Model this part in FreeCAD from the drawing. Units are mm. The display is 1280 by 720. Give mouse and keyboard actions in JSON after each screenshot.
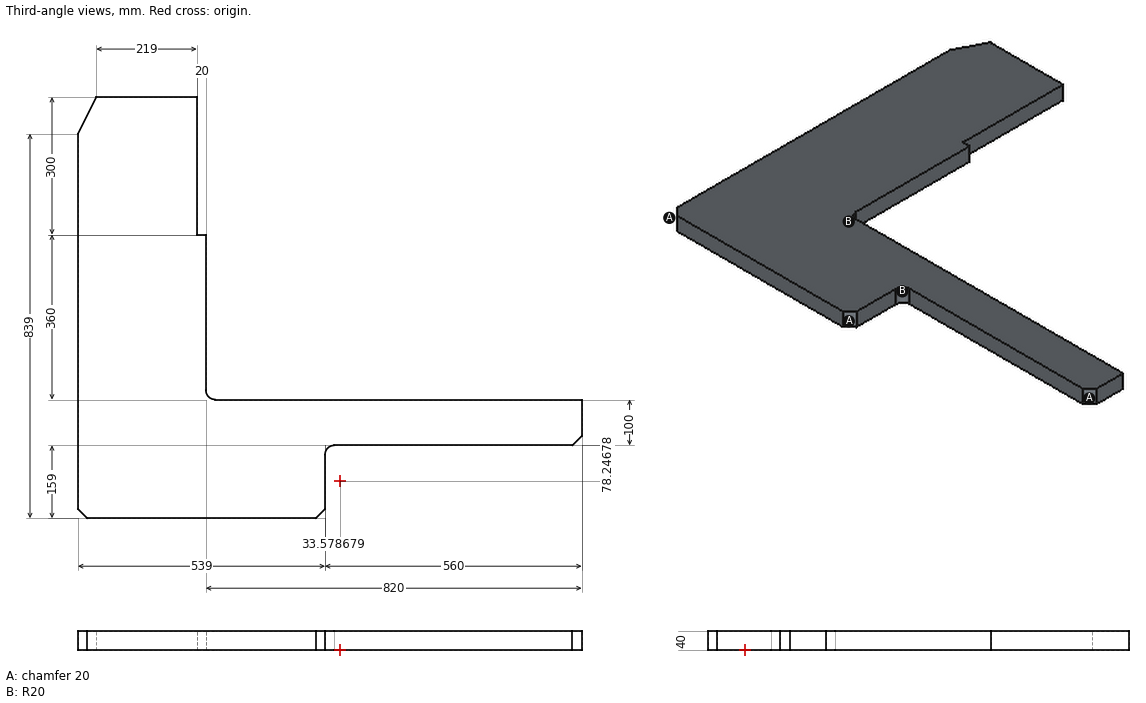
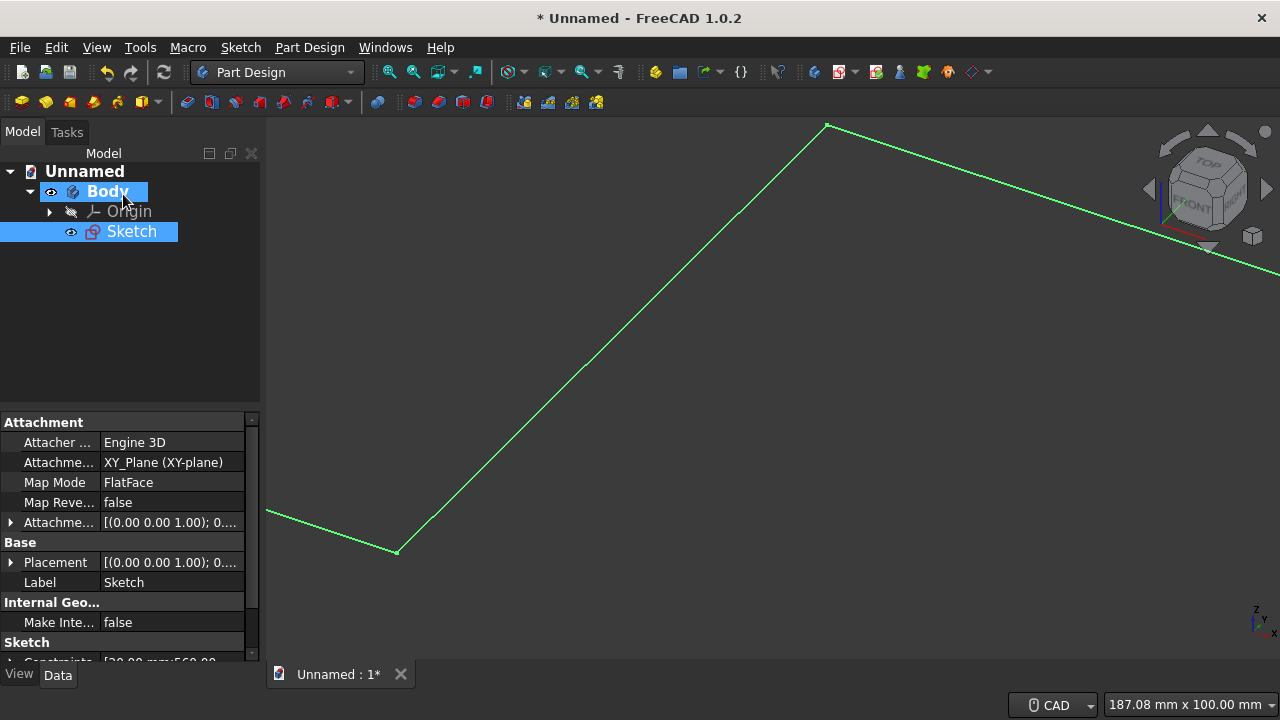
{"action": "left_click", "coordinate": [22, 102]}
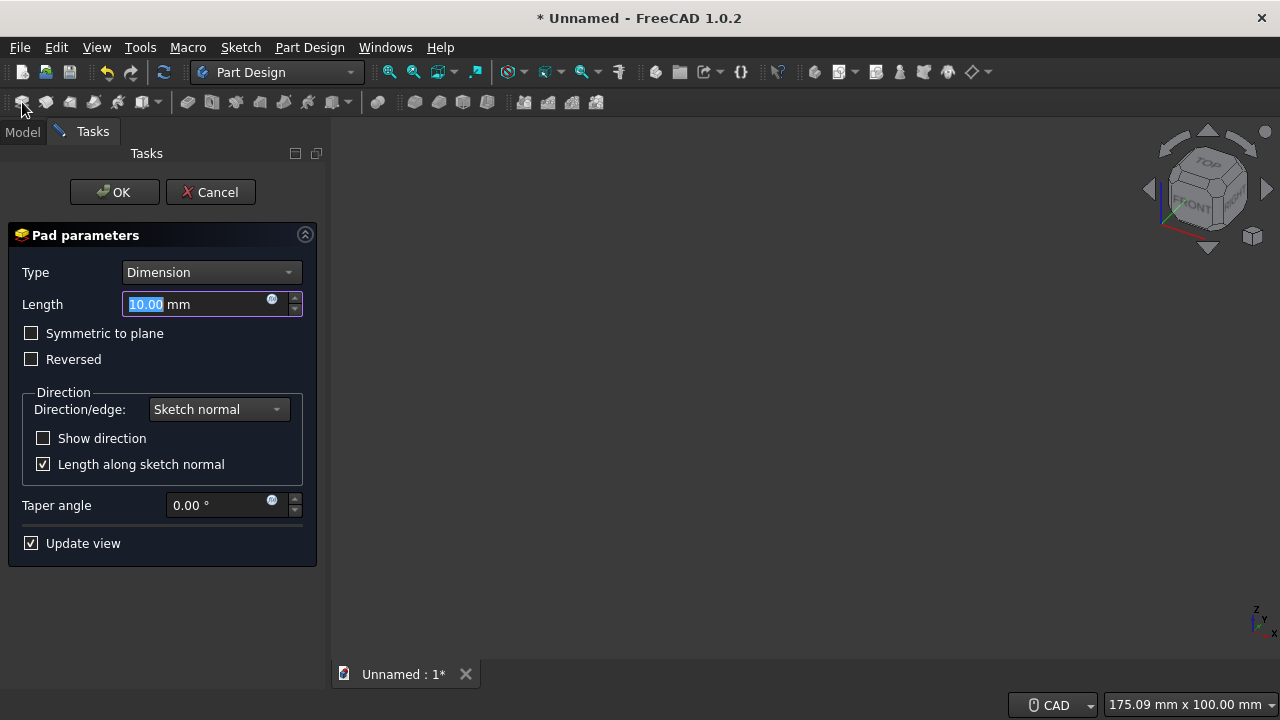
{"action": "type", "text": "40"}
{"action": "key", "text": "Tab"}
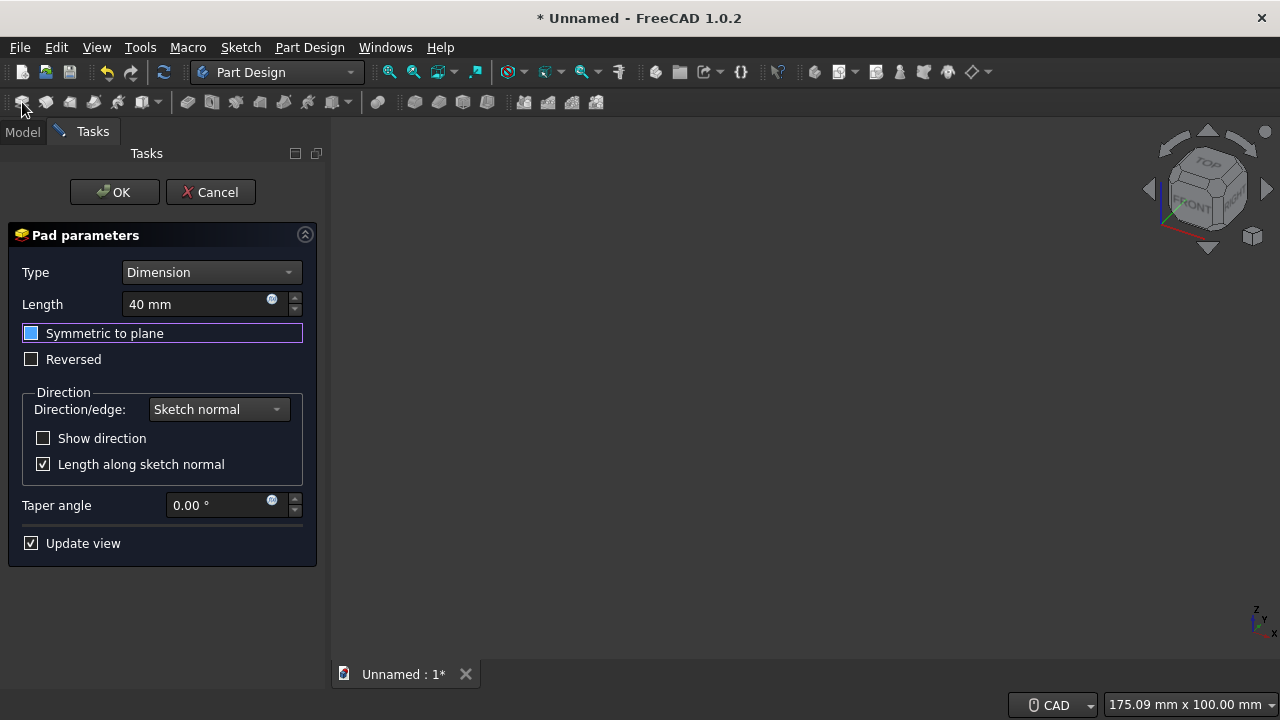
{"action": "left_click", "coordinate": [115, 192]}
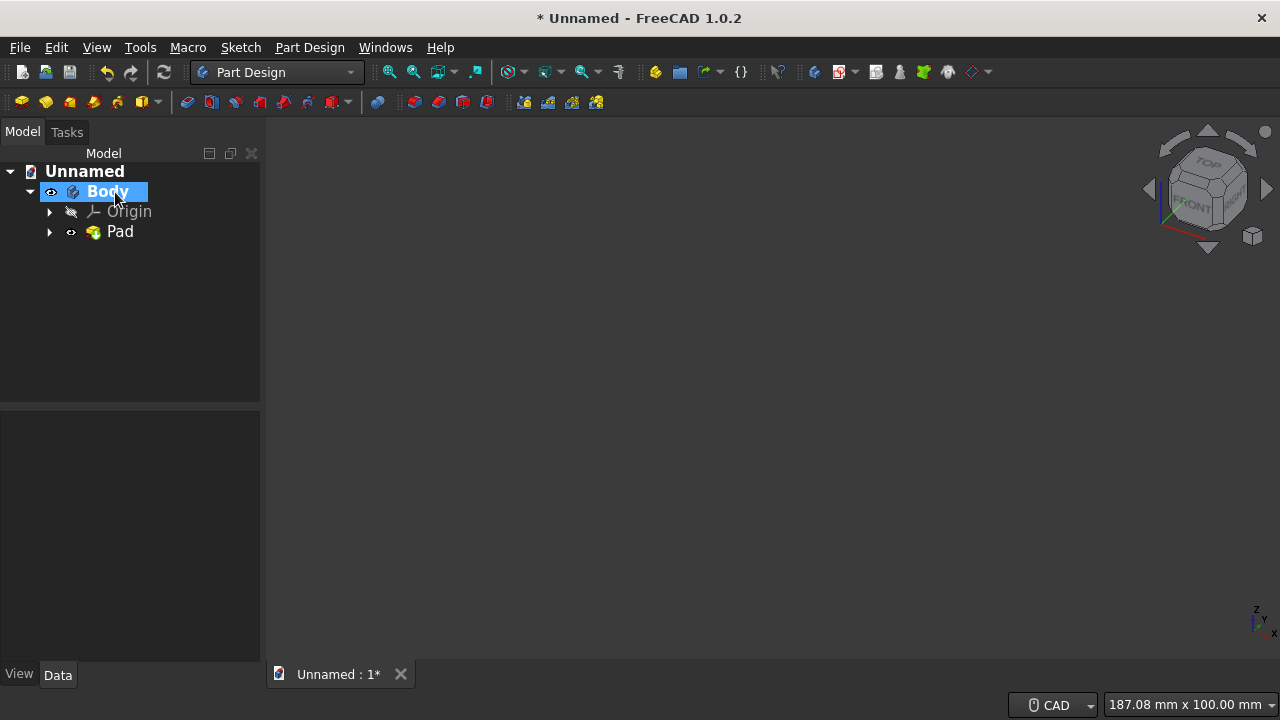
{"action": "left_click", "coordinate": [390, 72]}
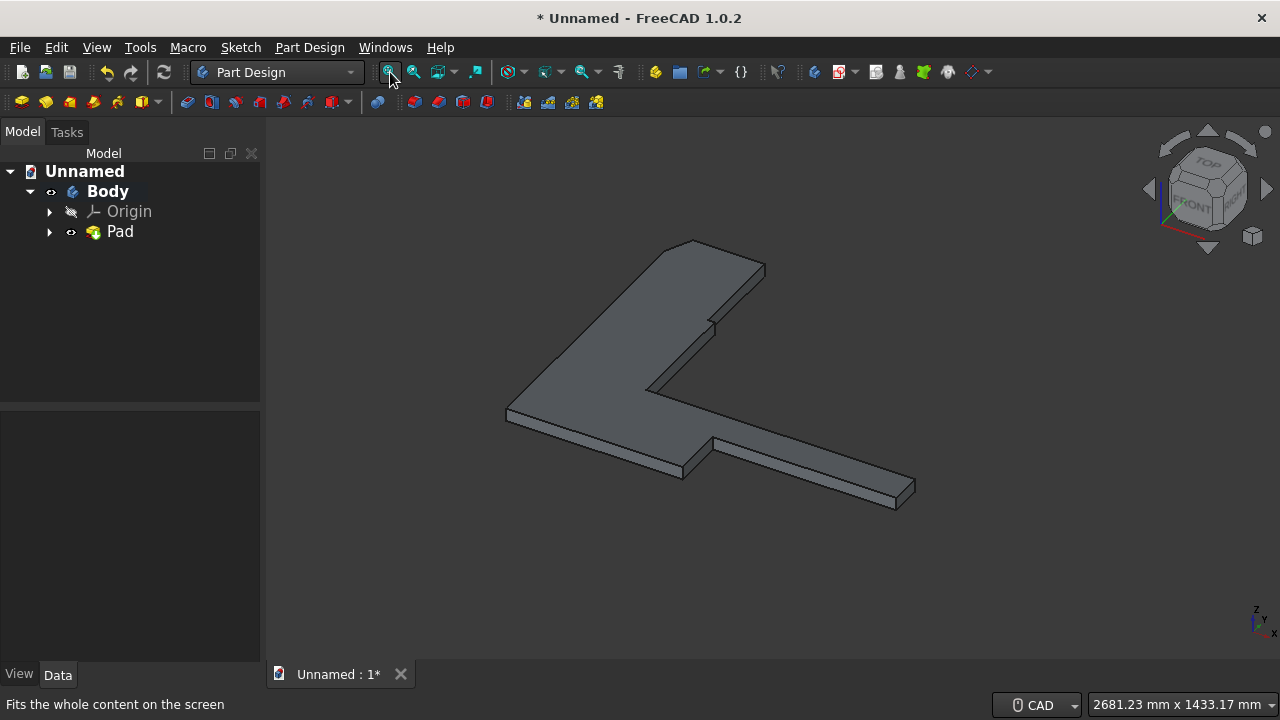
{"action": "left_click", "coordinate": [896, 503]}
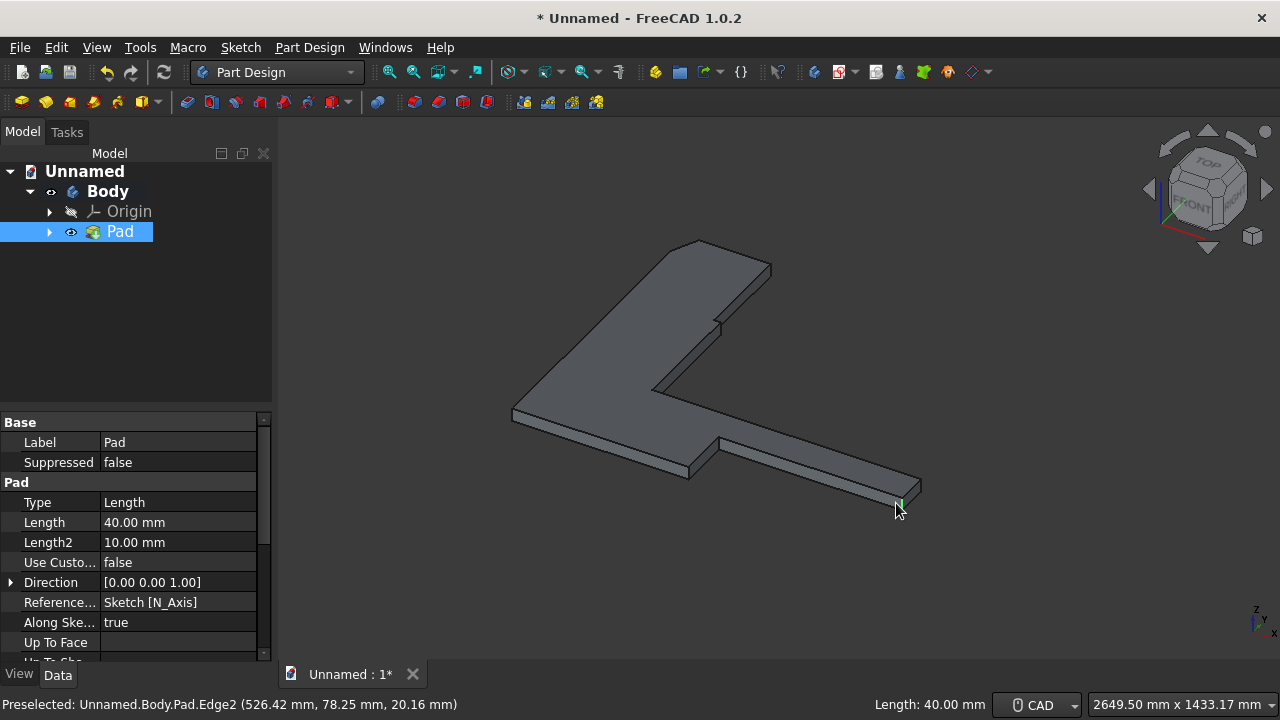
{"action": "left_click", "coordinate": [689, 472], "text": "ctrl"}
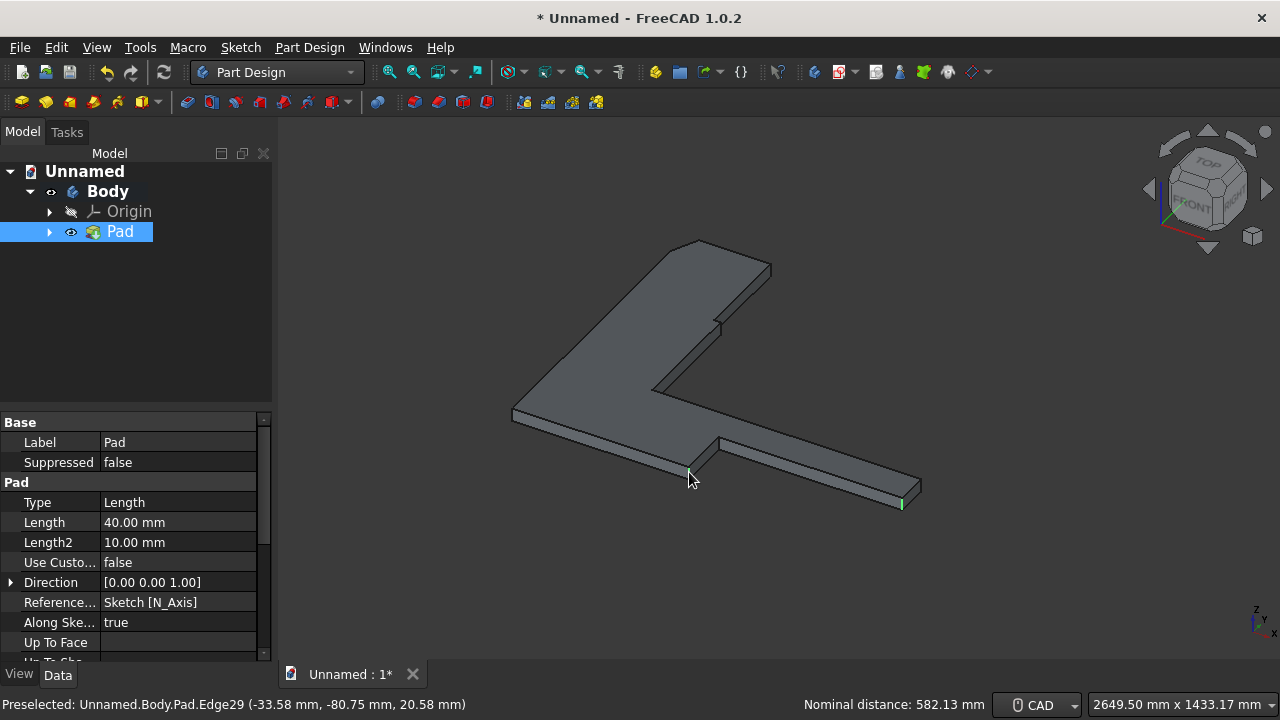
{"action": "scroll", "coordinate": [512, 414], "scroll_direction": "up", "scroll_amount": 5}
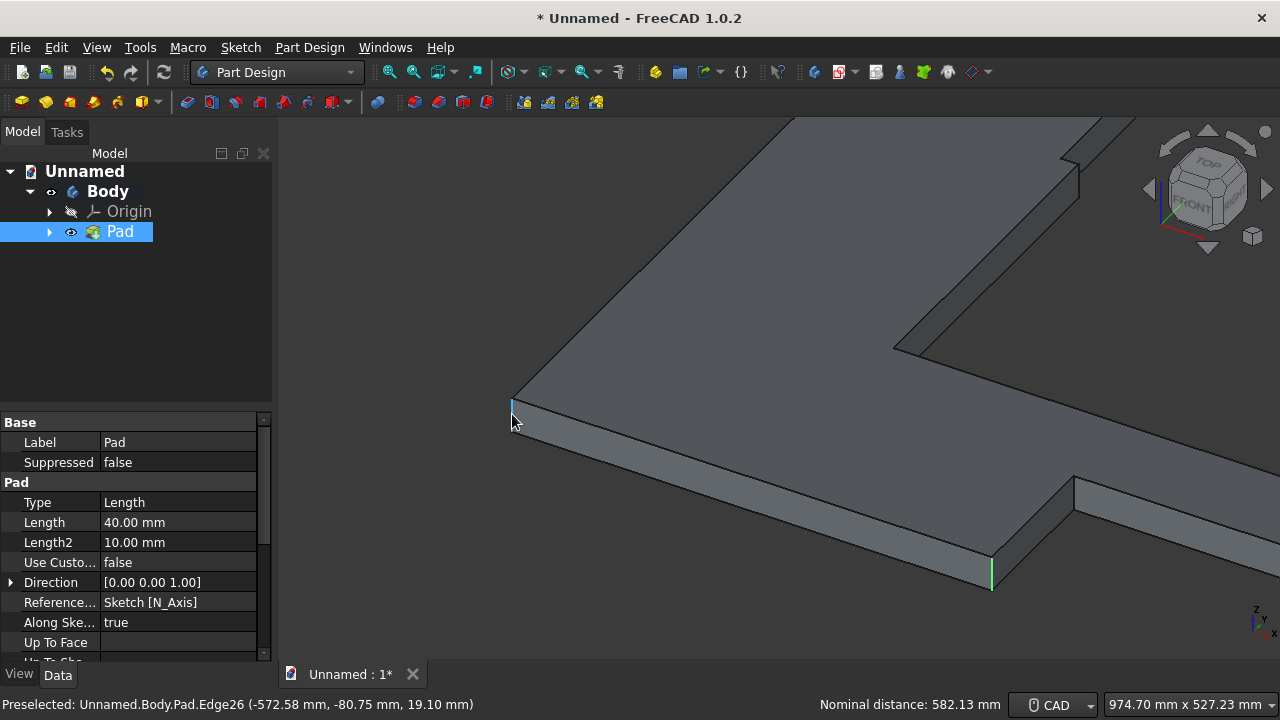
{"action": "key", "text": "v f"}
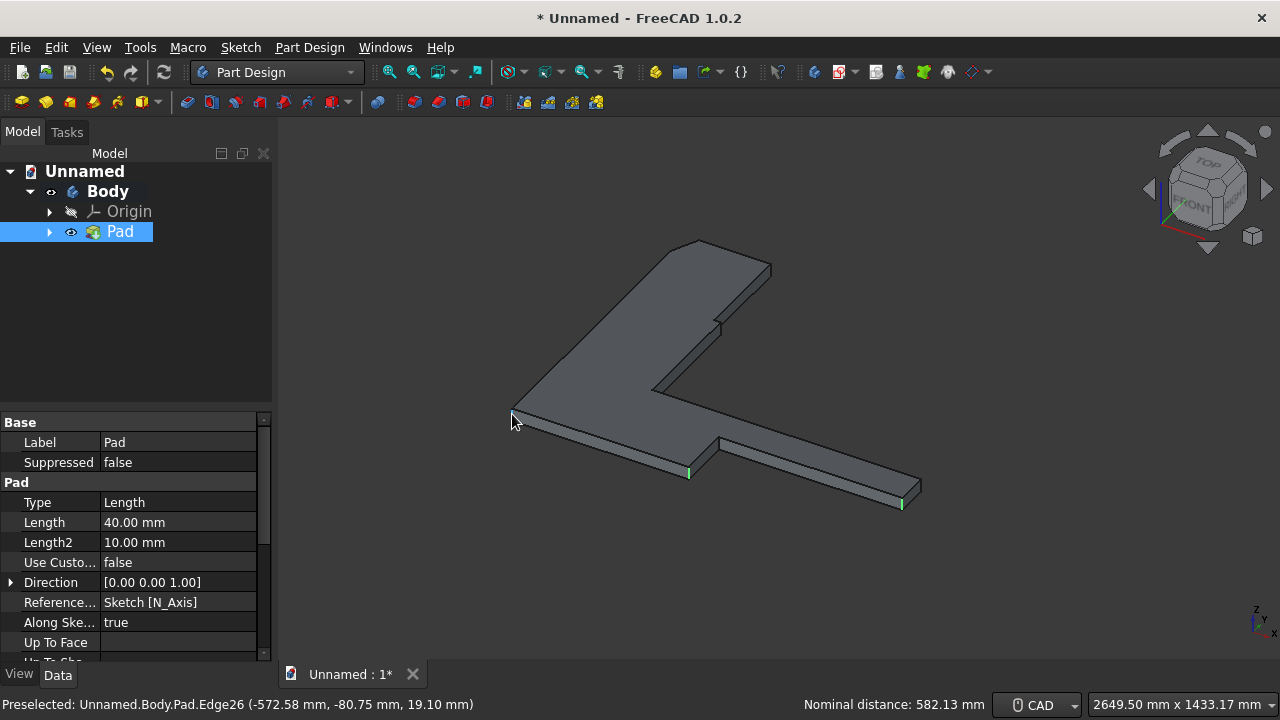
{"action": "key", "text": "0"}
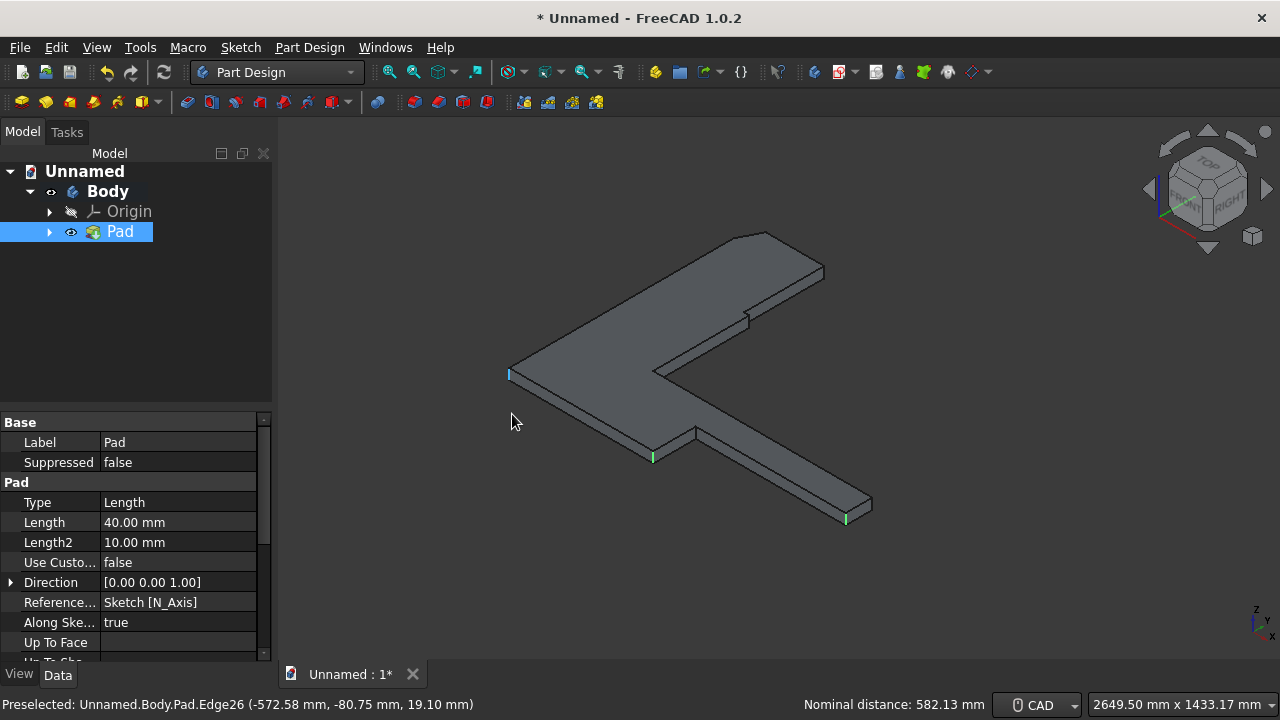
{"action": "scroll", "coordinate": [509, 373], "scroll_direction": "up", "scroll_amount": 5}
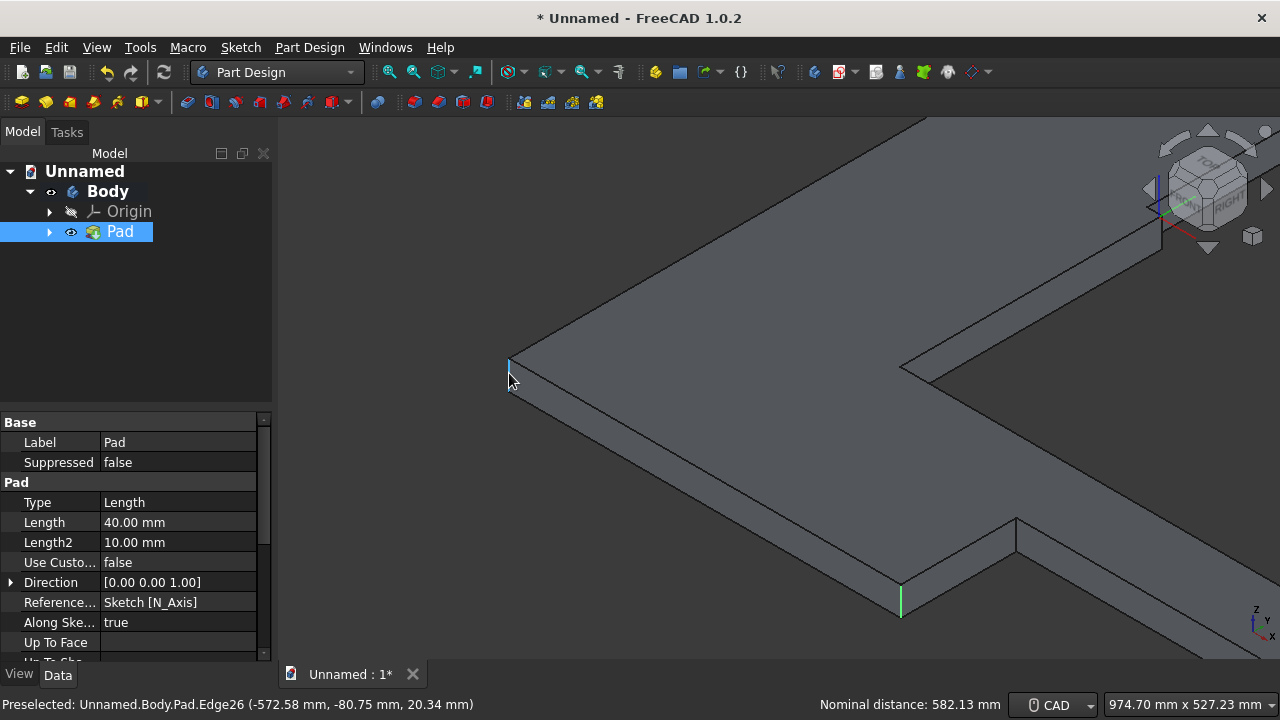
{"action": "key", "text": "v f"}